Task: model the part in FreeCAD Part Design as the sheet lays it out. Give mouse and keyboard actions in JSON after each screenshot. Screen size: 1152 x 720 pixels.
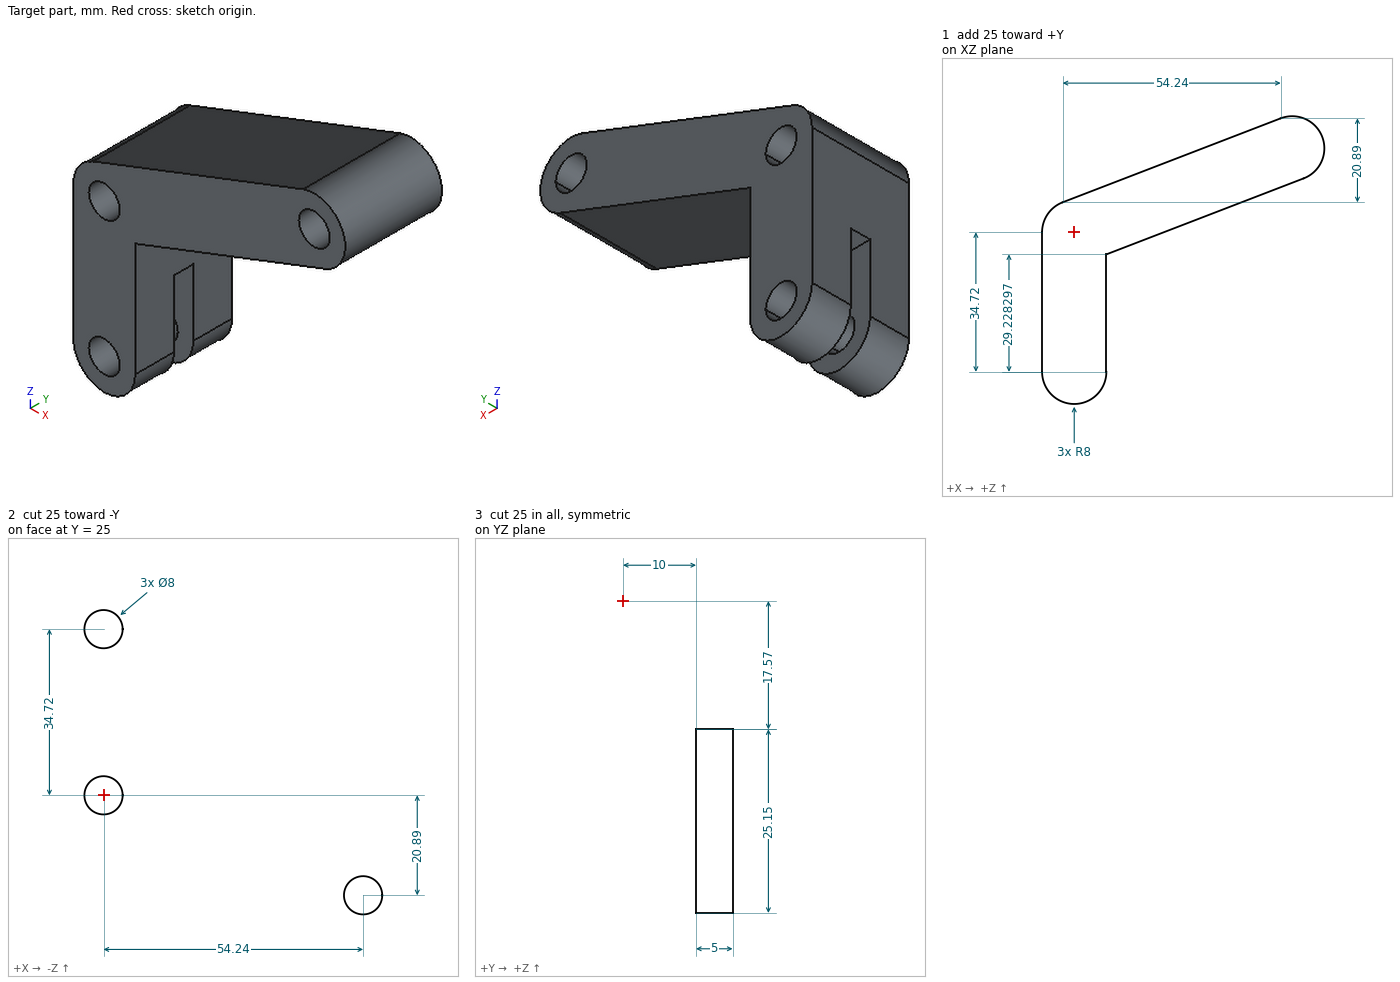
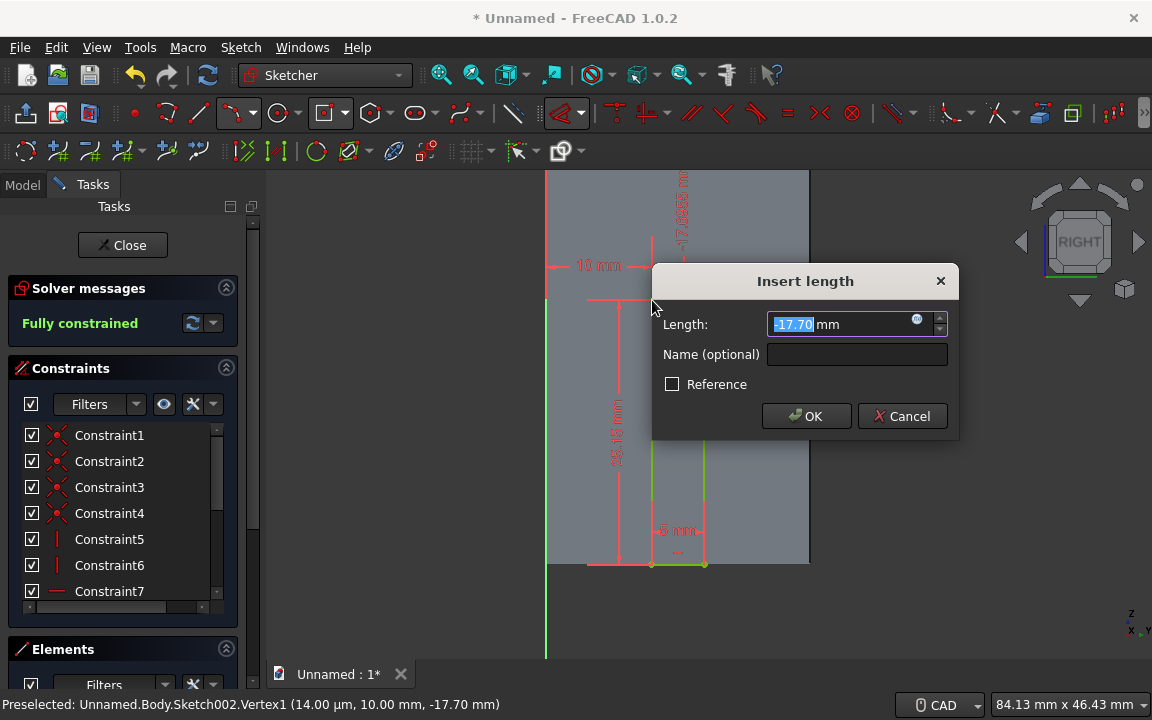
{"action": "type", "text": "-17.57"}
{"action": "key", "text": "Return"}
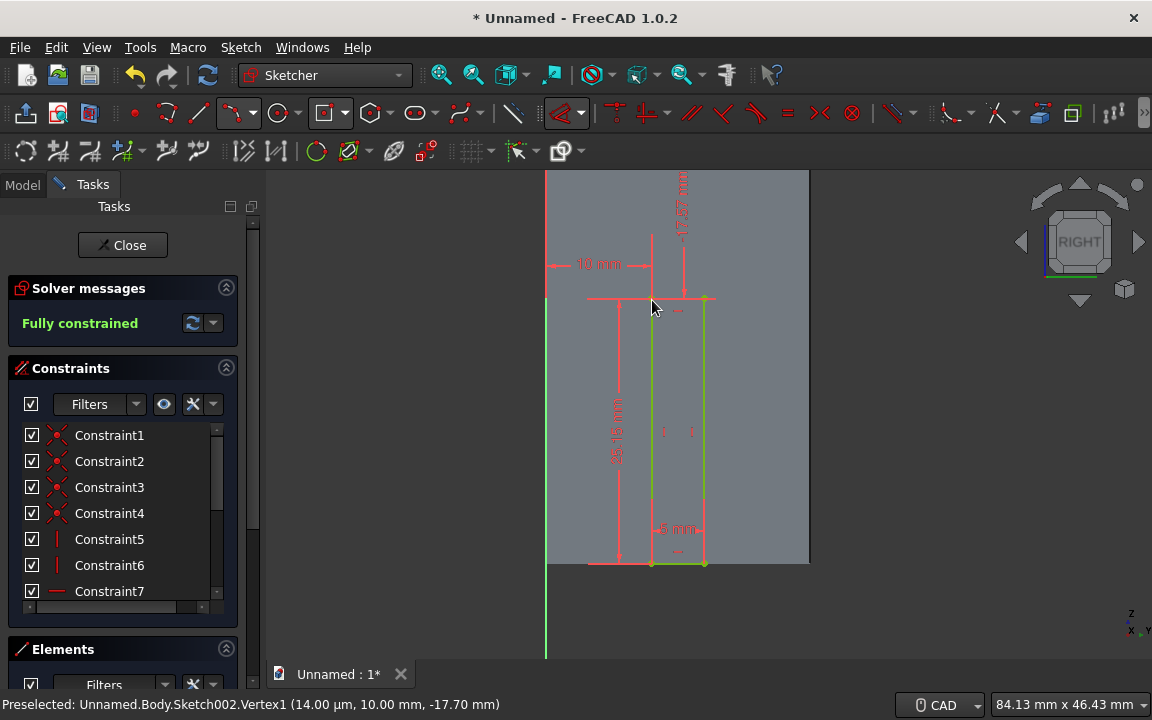
{"action": "left_click", "coordinate": [123, 245]}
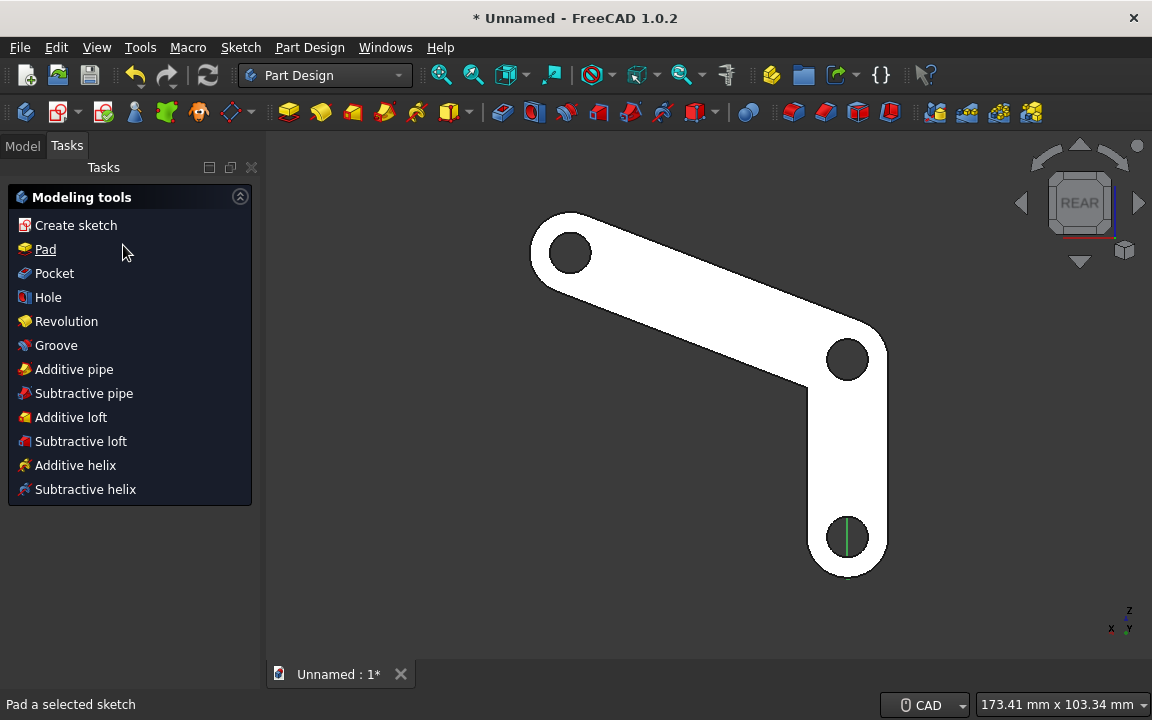
{"action": "left_click", "coordinate": [504, 112]}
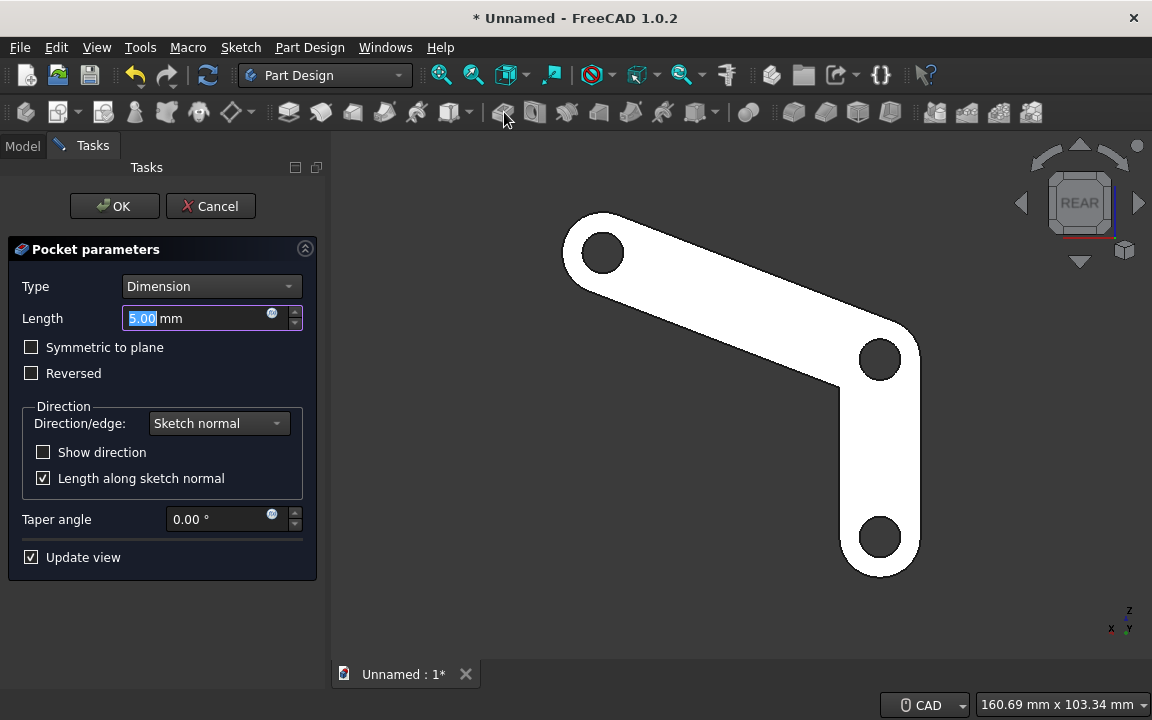
{"action": "type", "text": "25"}
{"action": "key", "text": "Tab"}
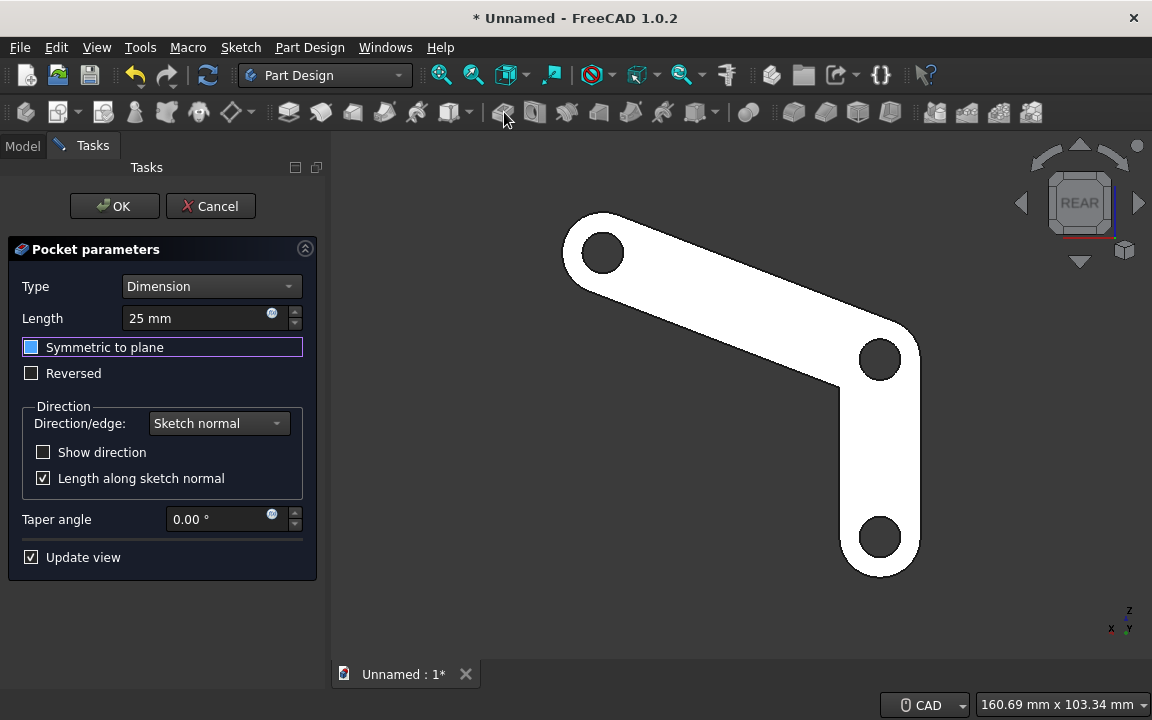
{"action": "left_click", "coordinate": [30, 347]}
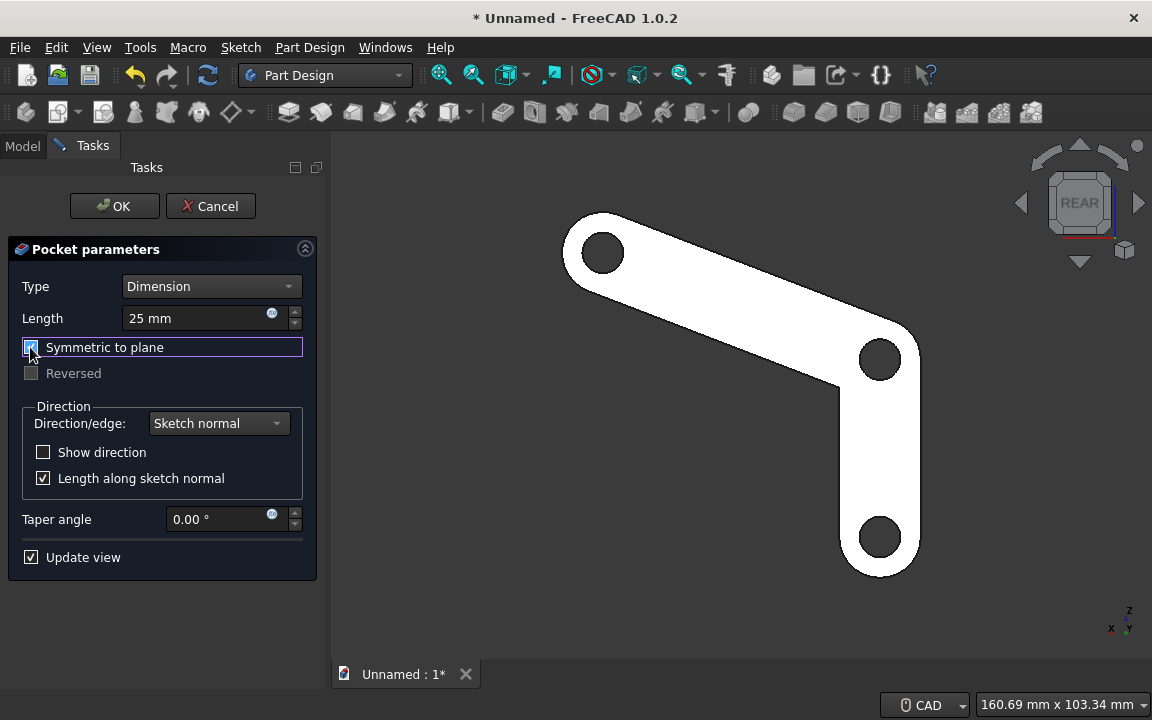
{"action": "left_click", "coordinate": [115, 206]}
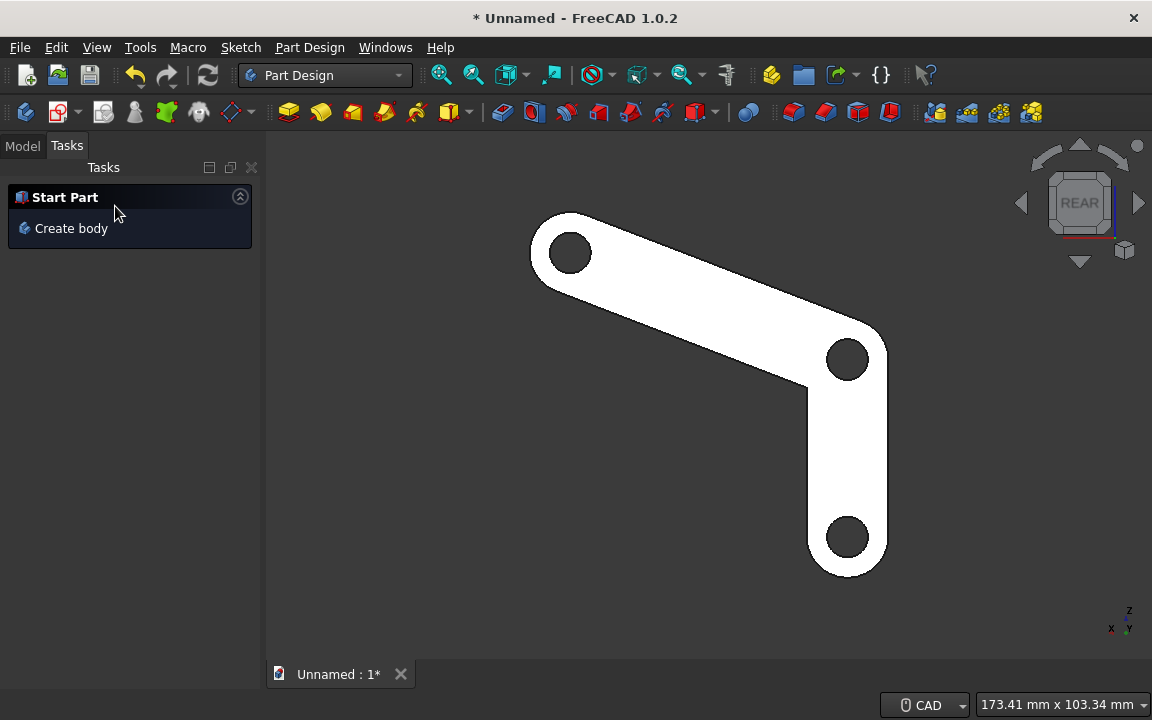
{"action": "key", "text": "0"}